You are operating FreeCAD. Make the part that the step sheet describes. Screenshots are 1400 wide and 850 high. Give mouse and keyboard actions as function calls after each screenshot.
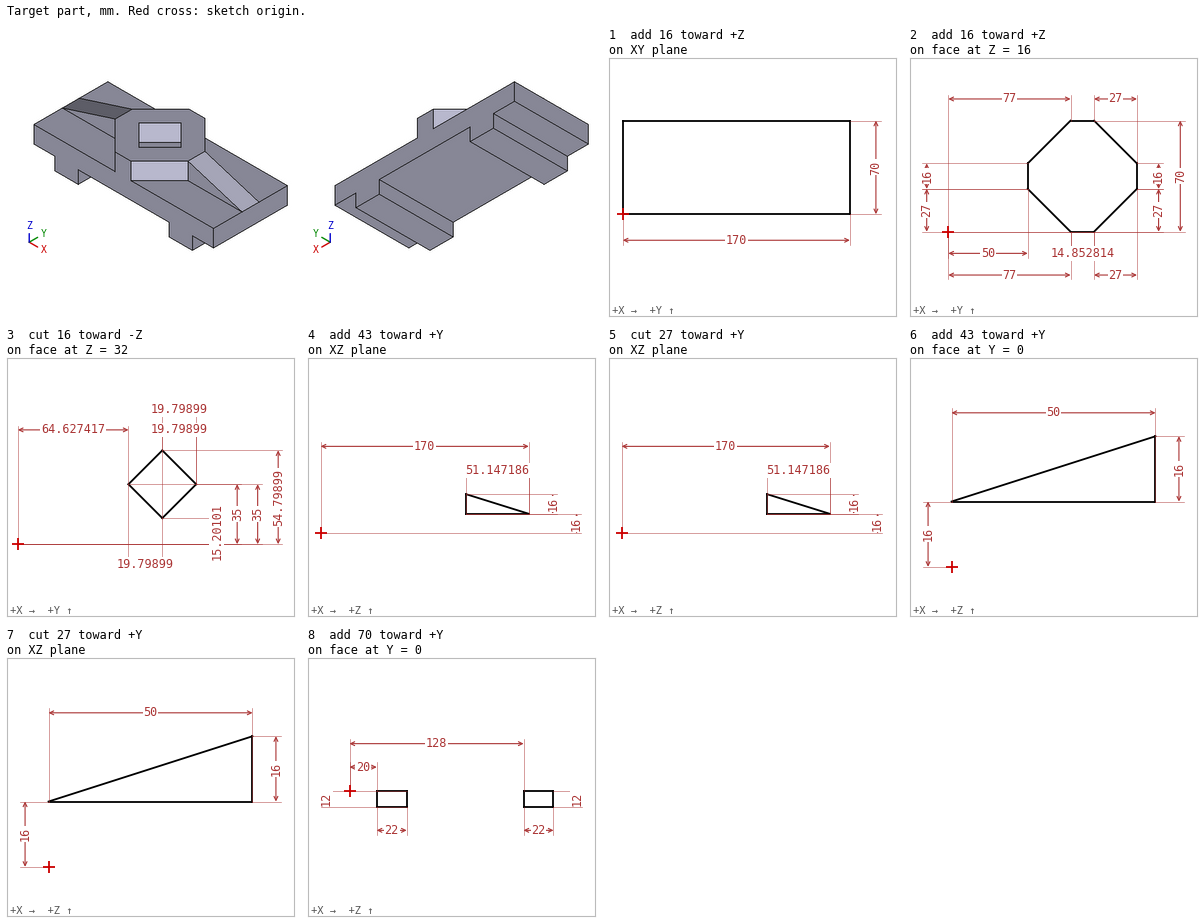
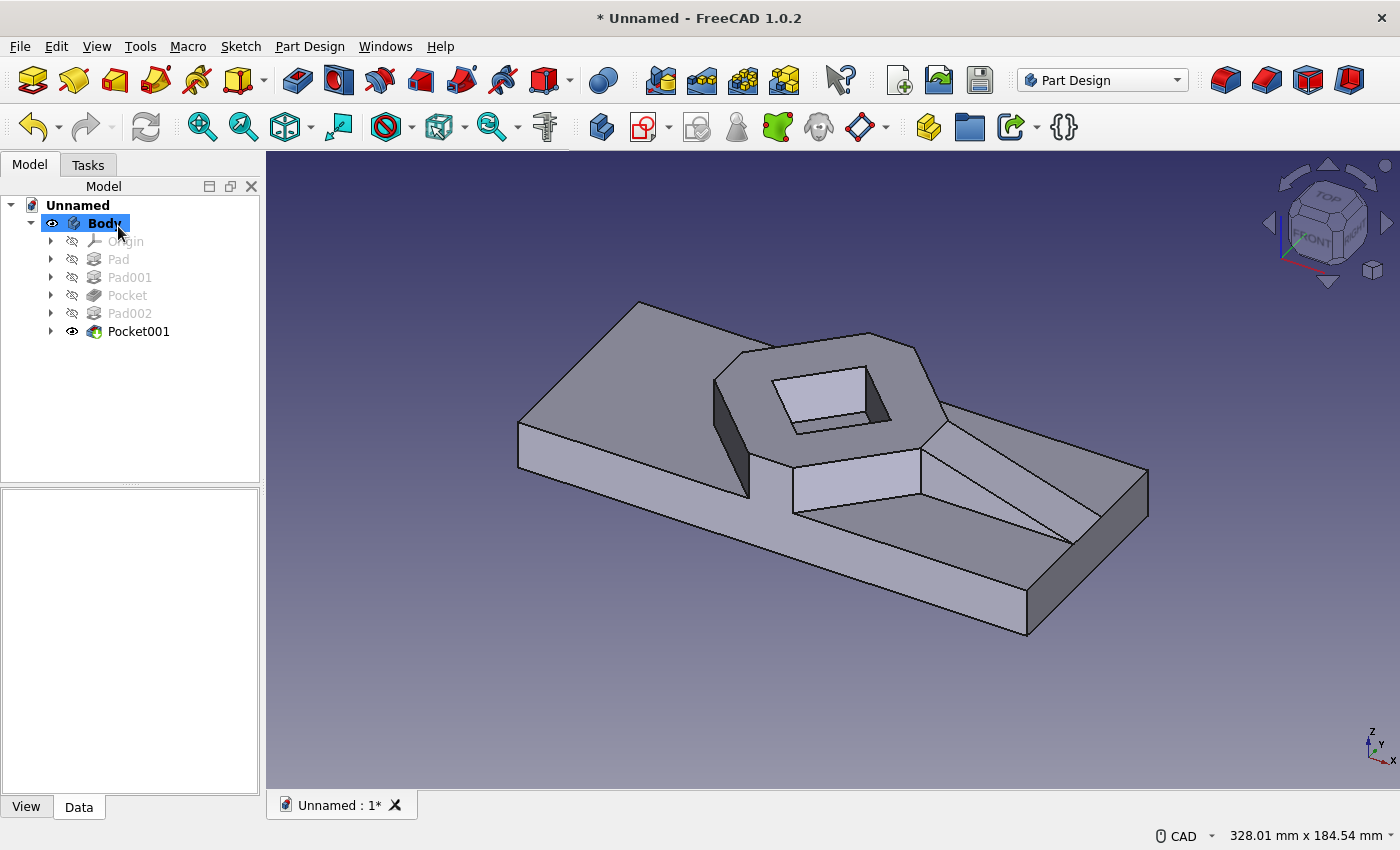
click(772, 518)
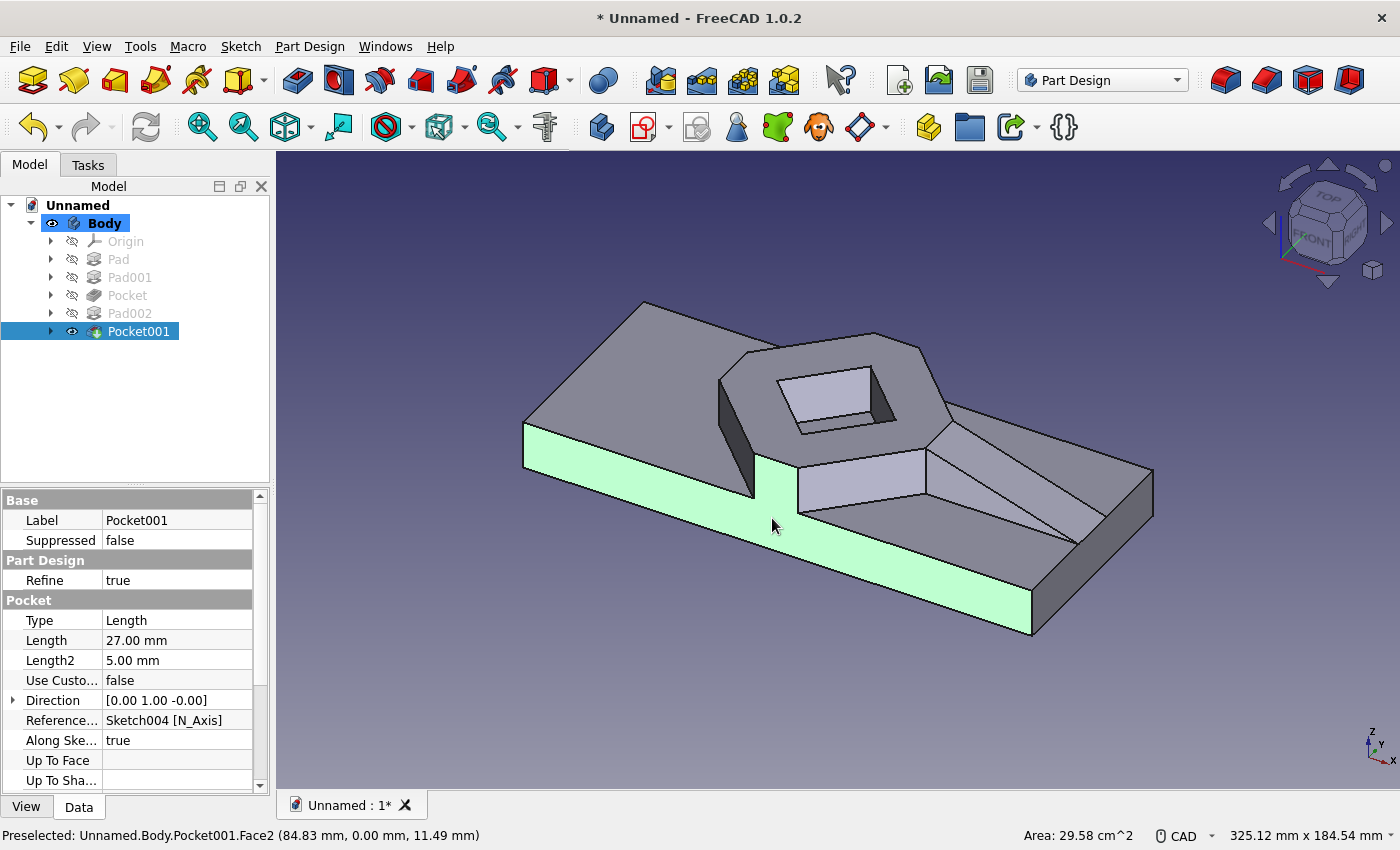
click(642, 128)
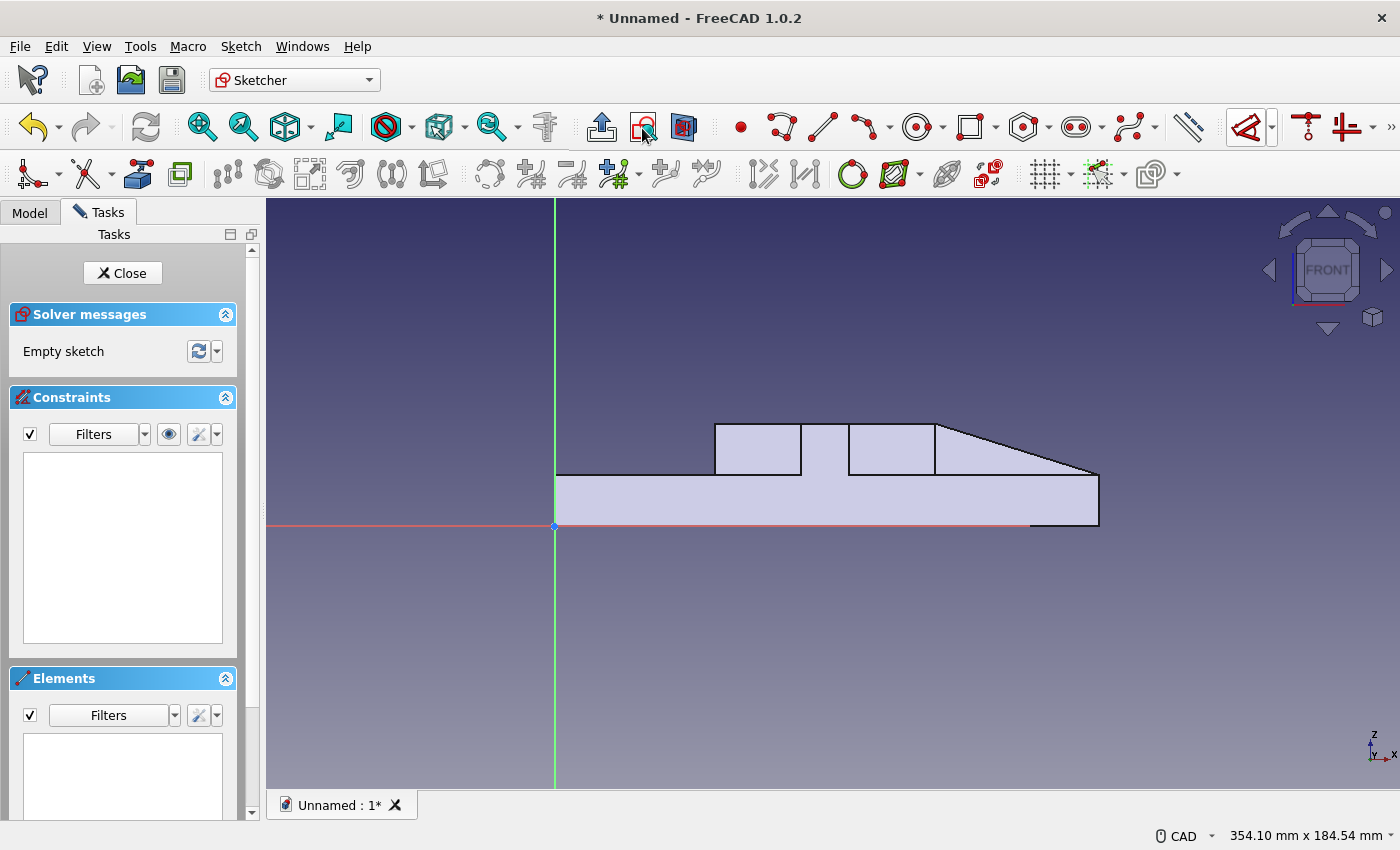
scroll(592, 469, up, 7)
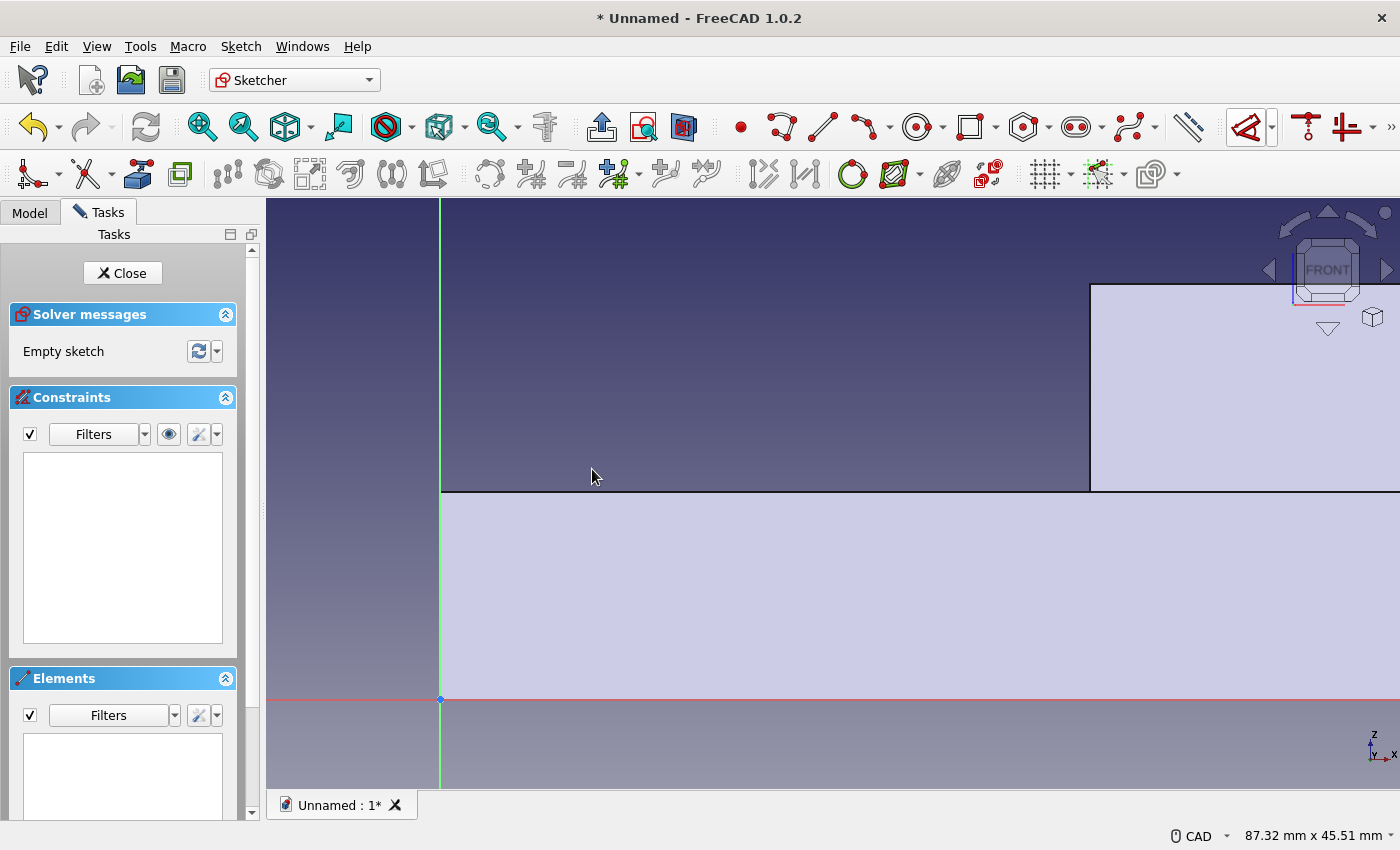
key(g)
key(m)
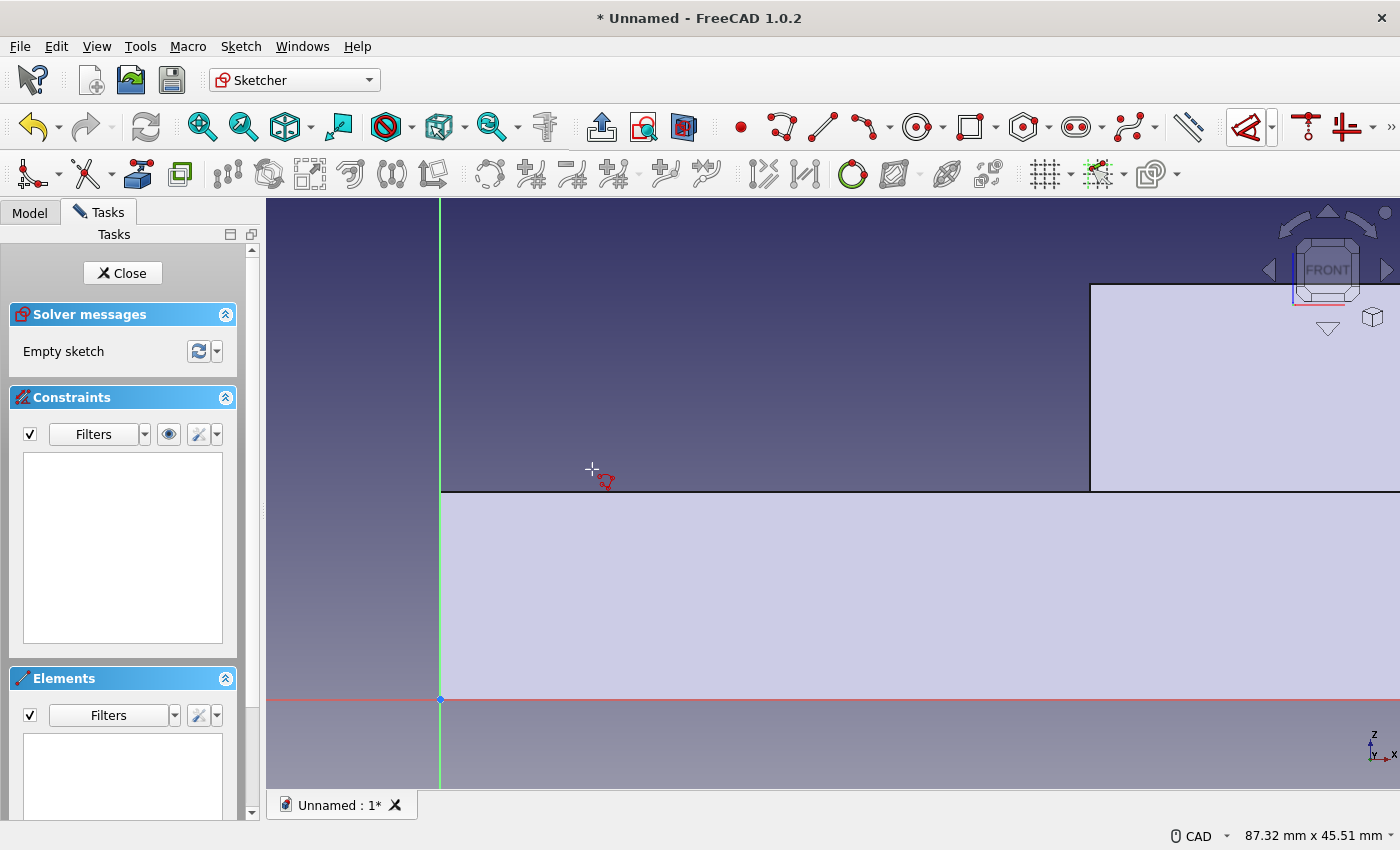
click(440, 492)
click(1090, 492)
click(1090, 284)
click(440, 493)
key(Escape)
key(Escape)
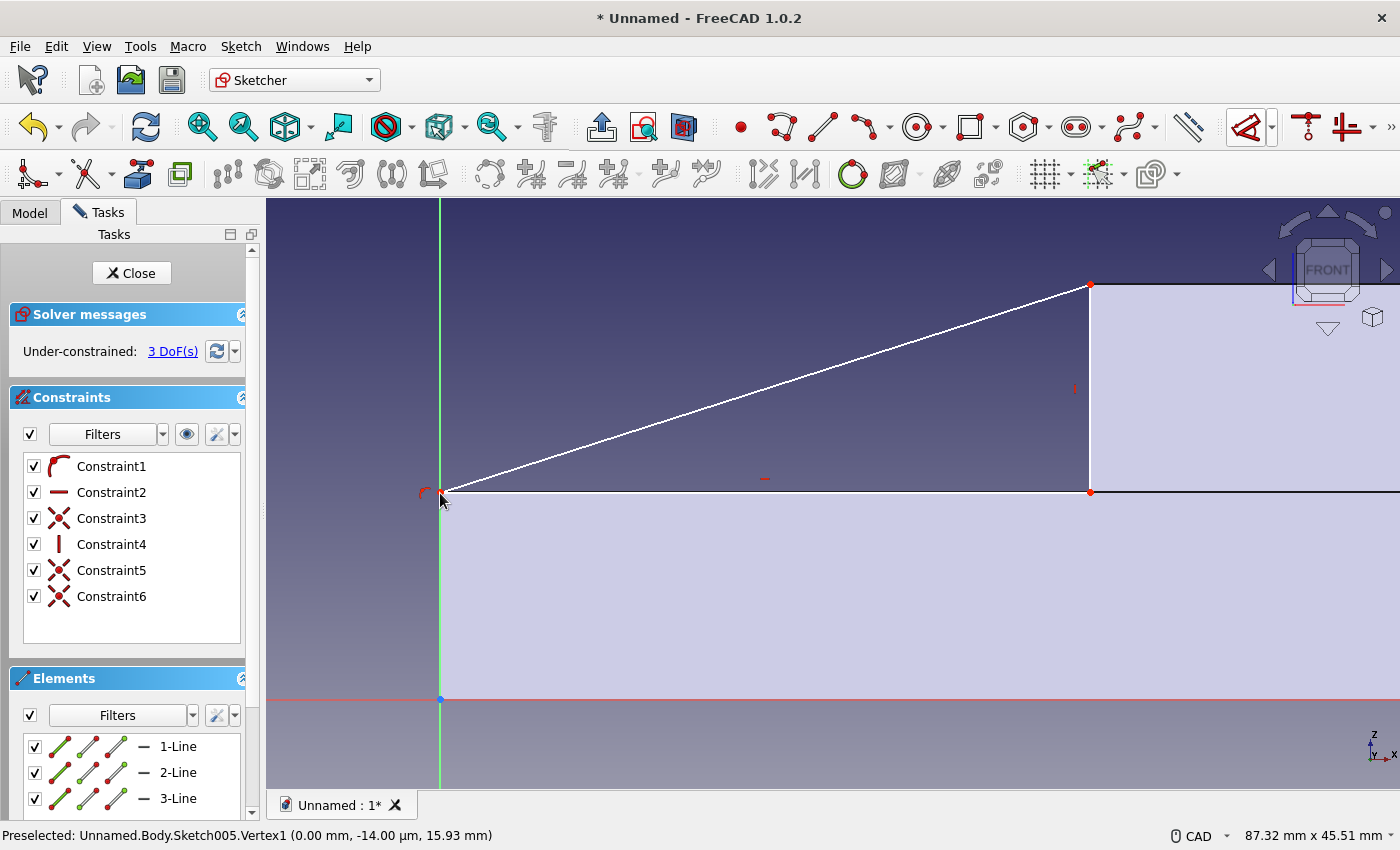
click(1246, 128)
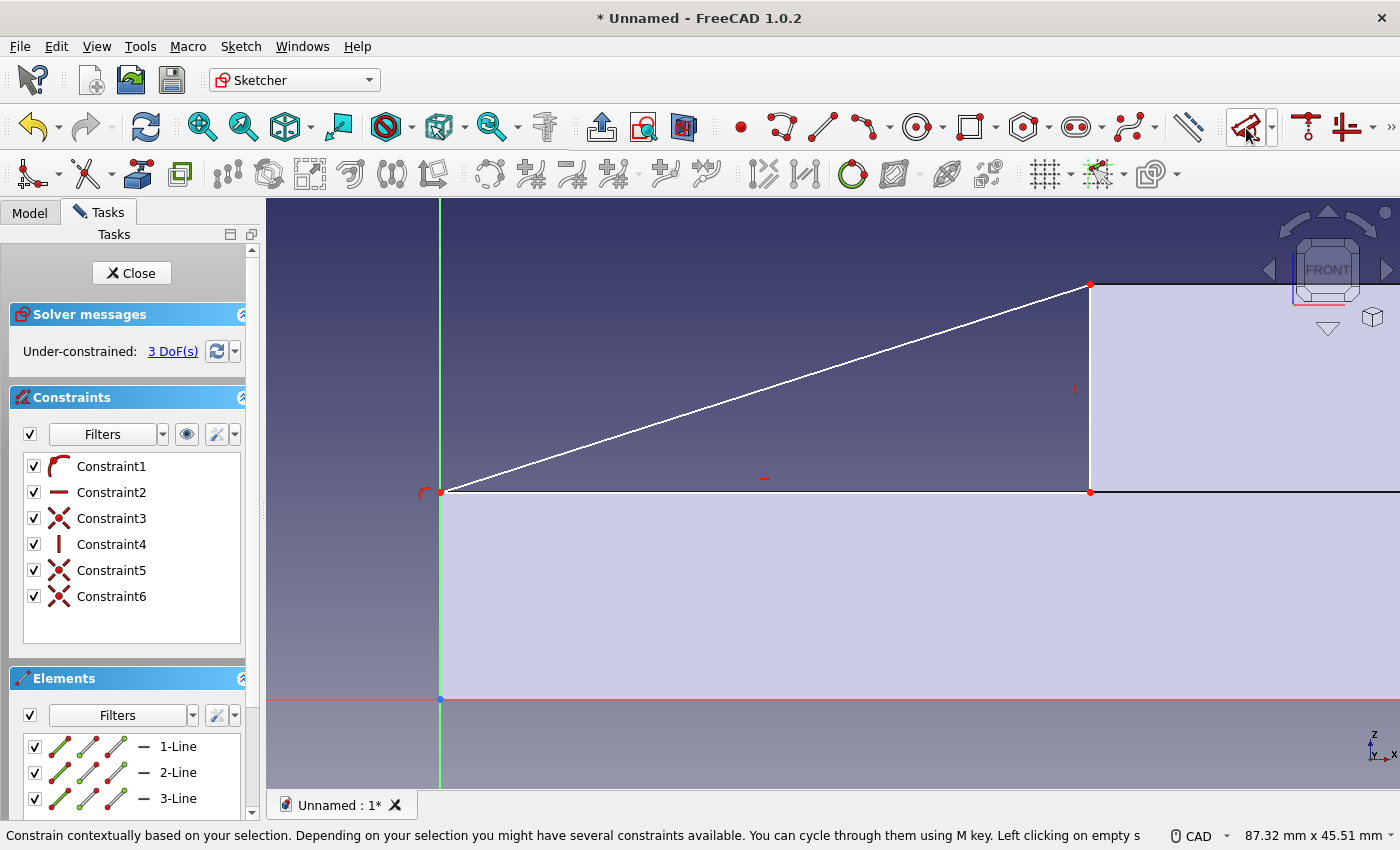
click(635, 493)
click(765, 527)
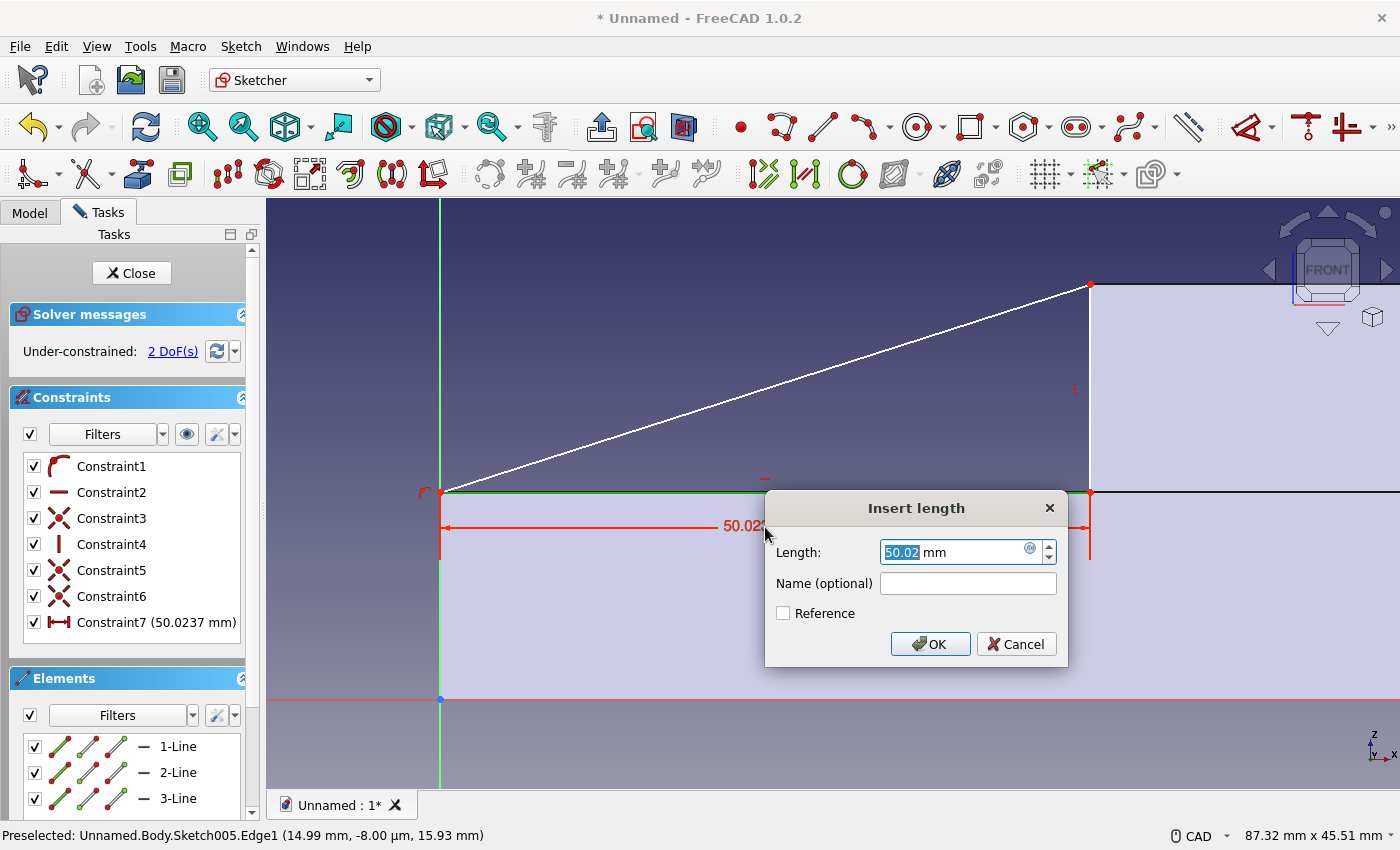
text(50)
key(Return)